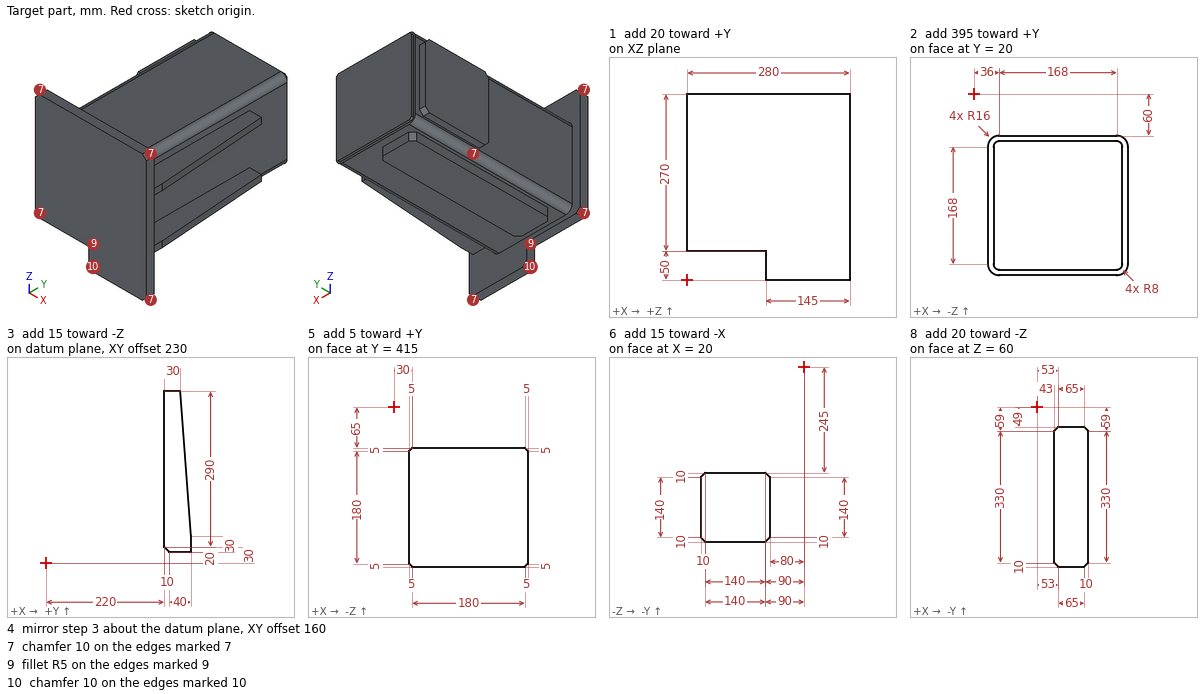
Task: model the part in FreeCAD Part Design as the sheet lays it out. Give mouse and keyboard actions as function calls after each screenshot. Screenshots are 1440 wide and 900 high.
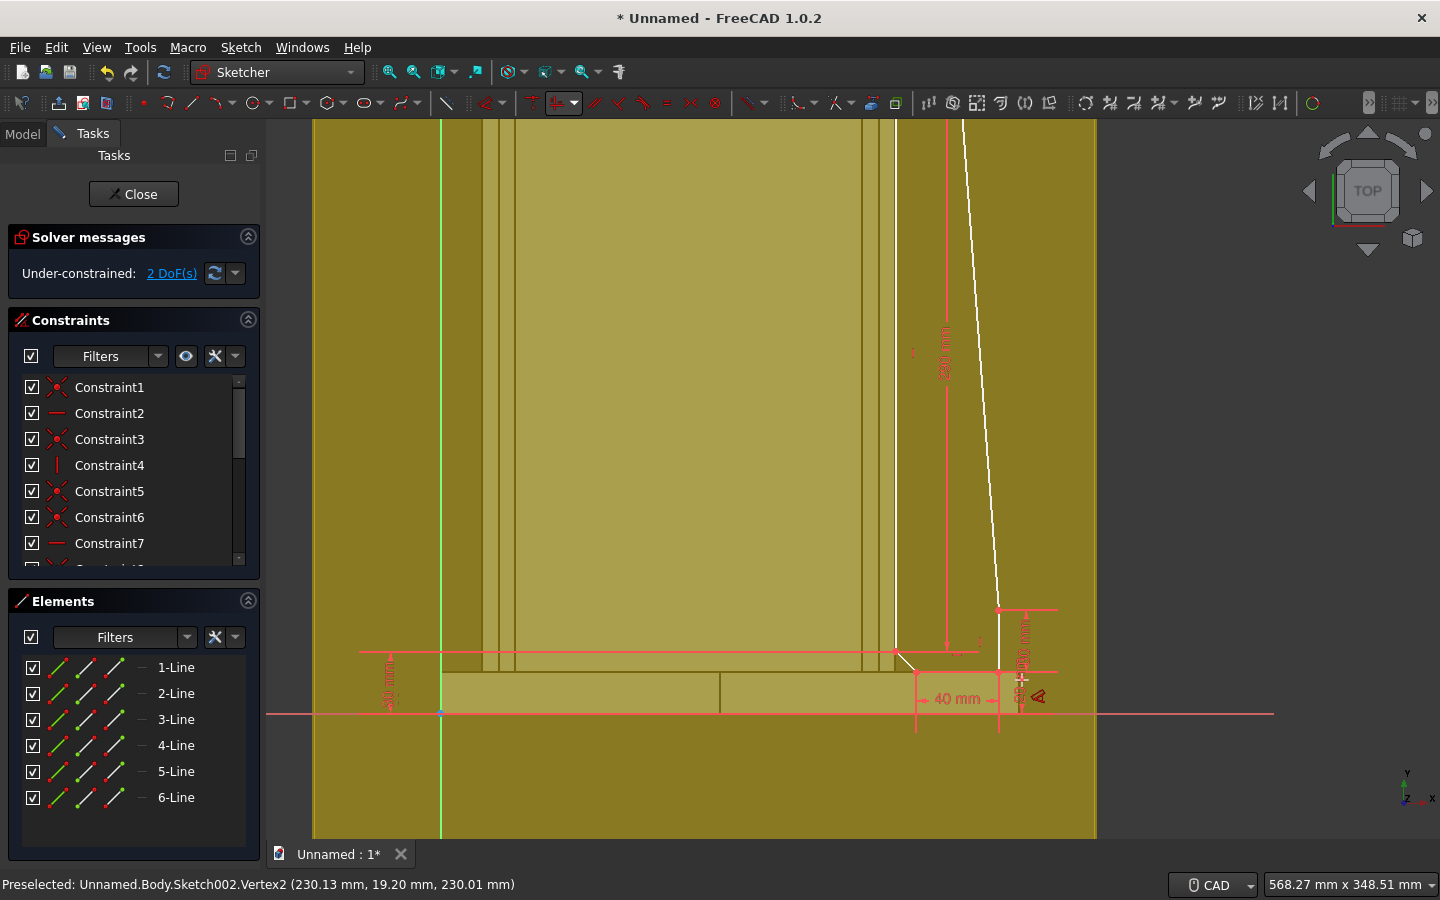
scroll(904, 660, up, 4)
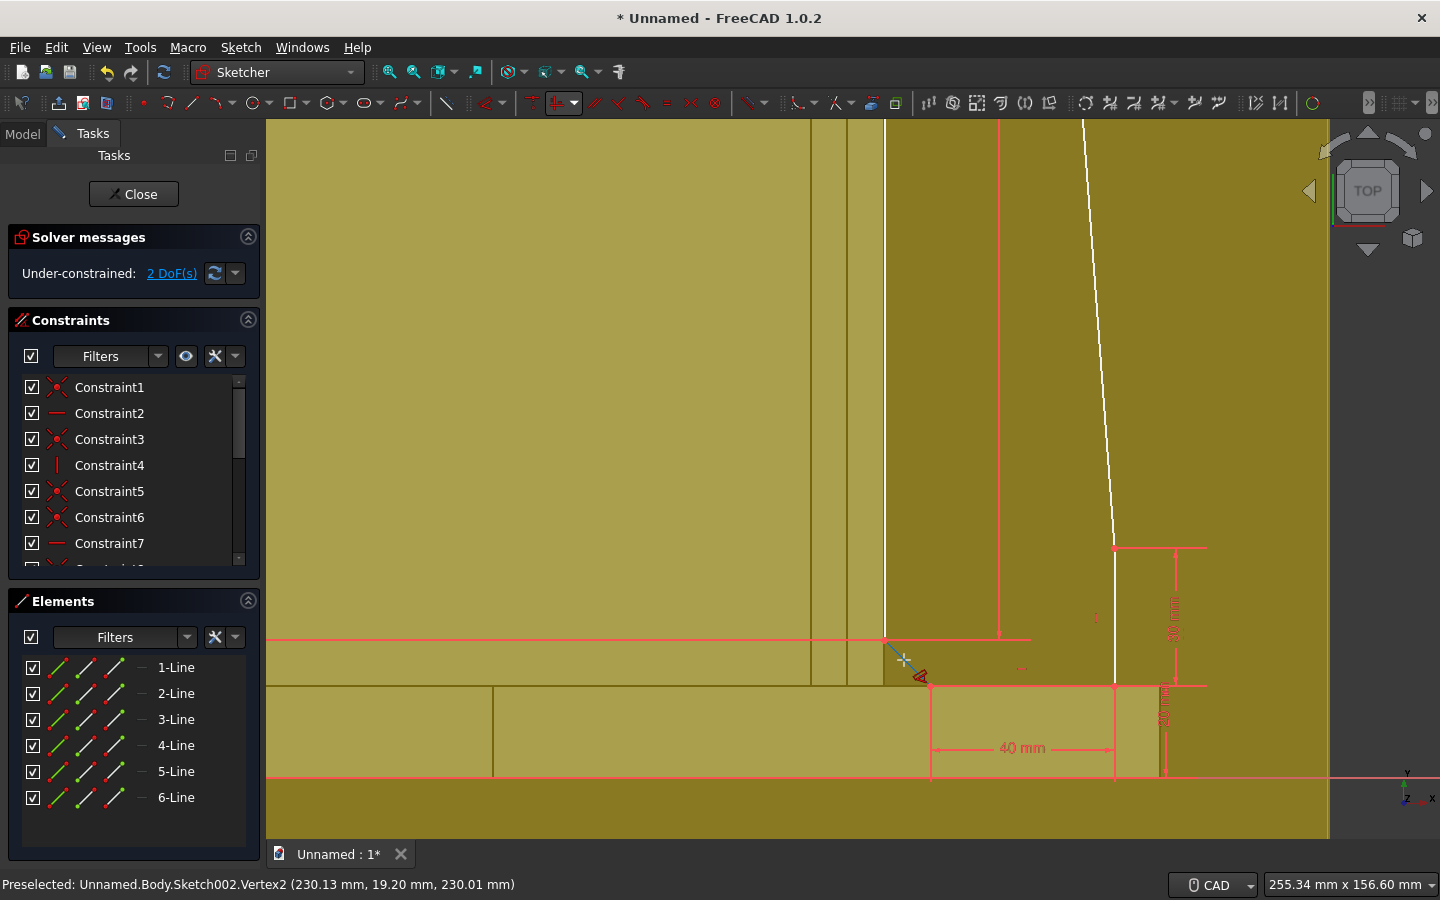
click(903, 659)
click(908, 720)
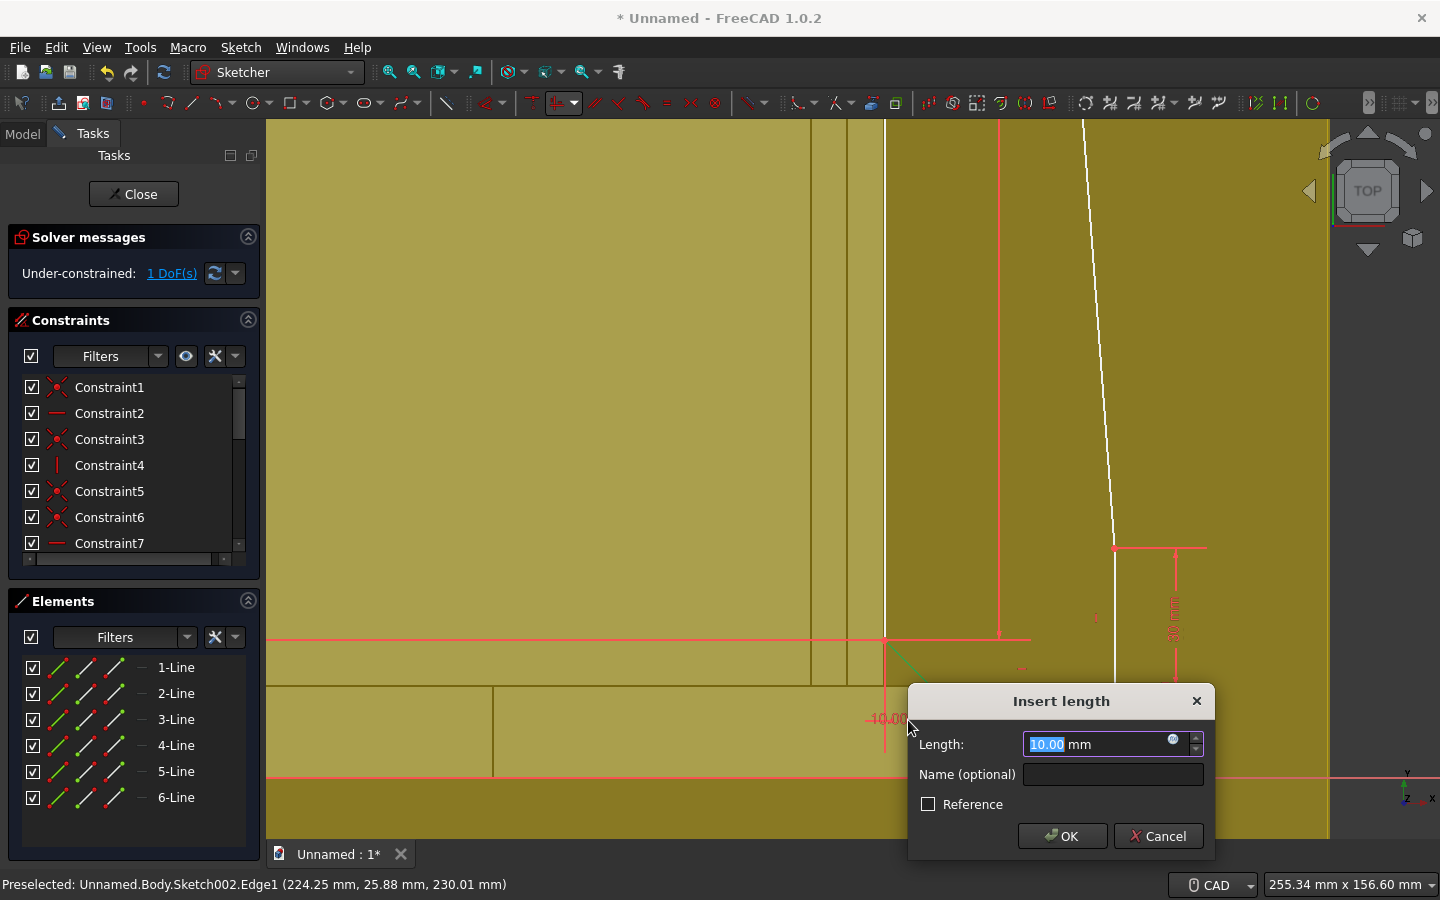
text(10)
key(Return)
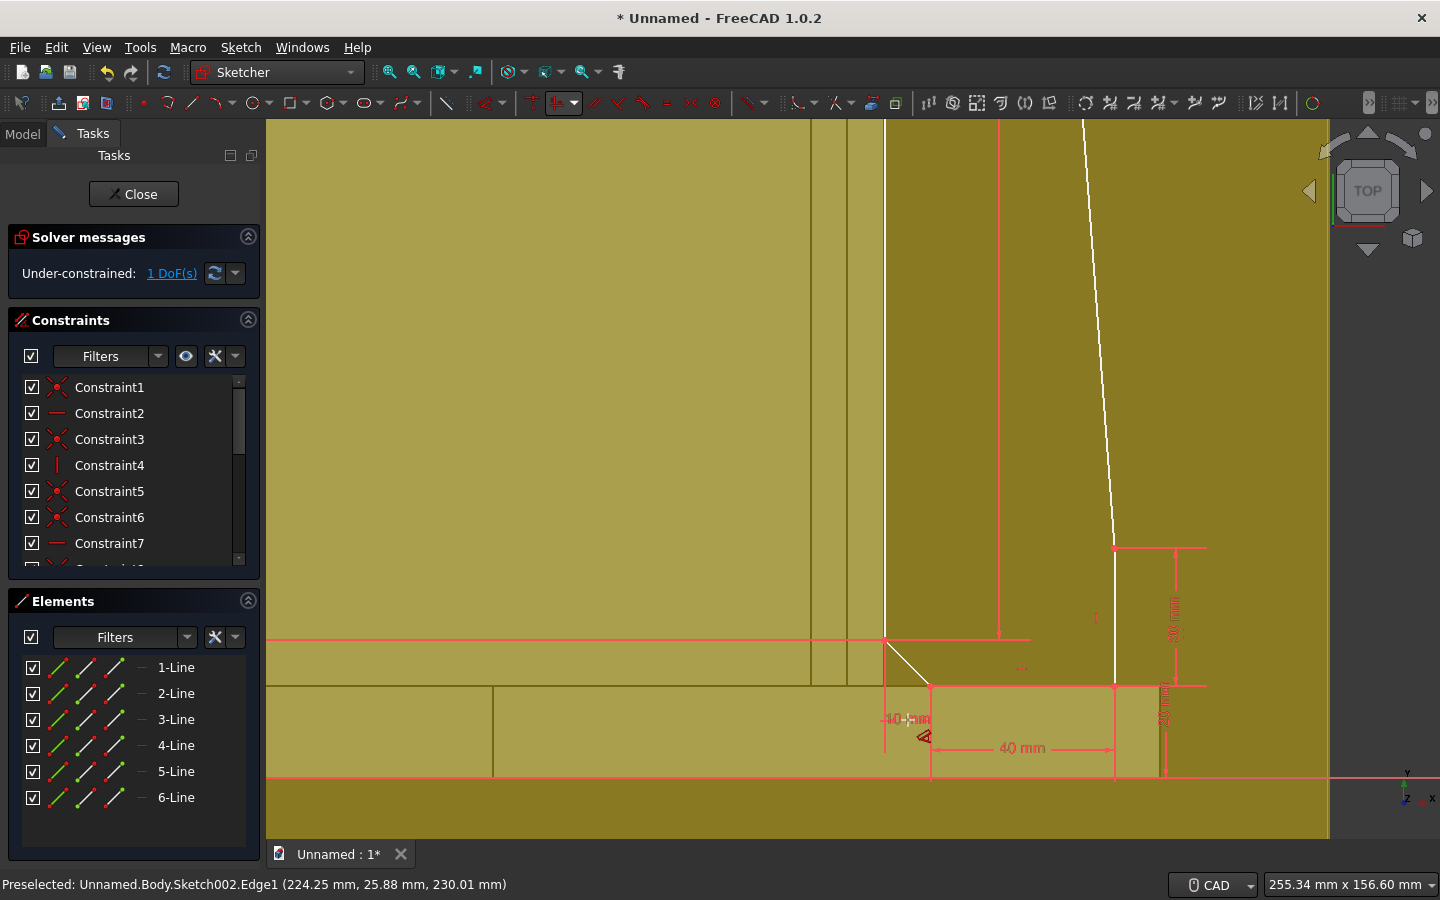
scroll(910, 667, down, 6)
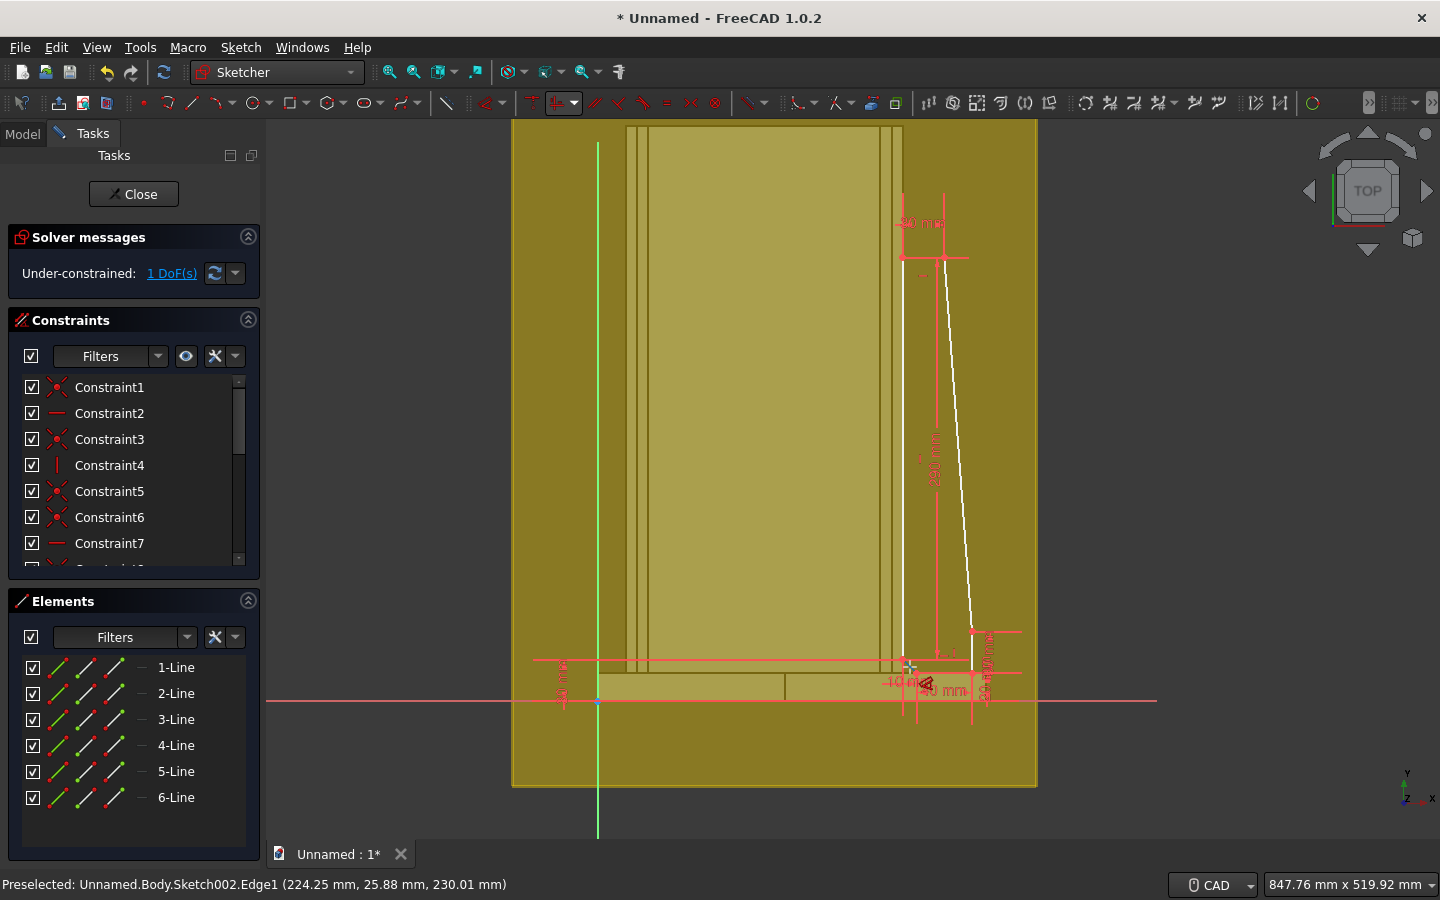
click(903, 660)
click(750, 735)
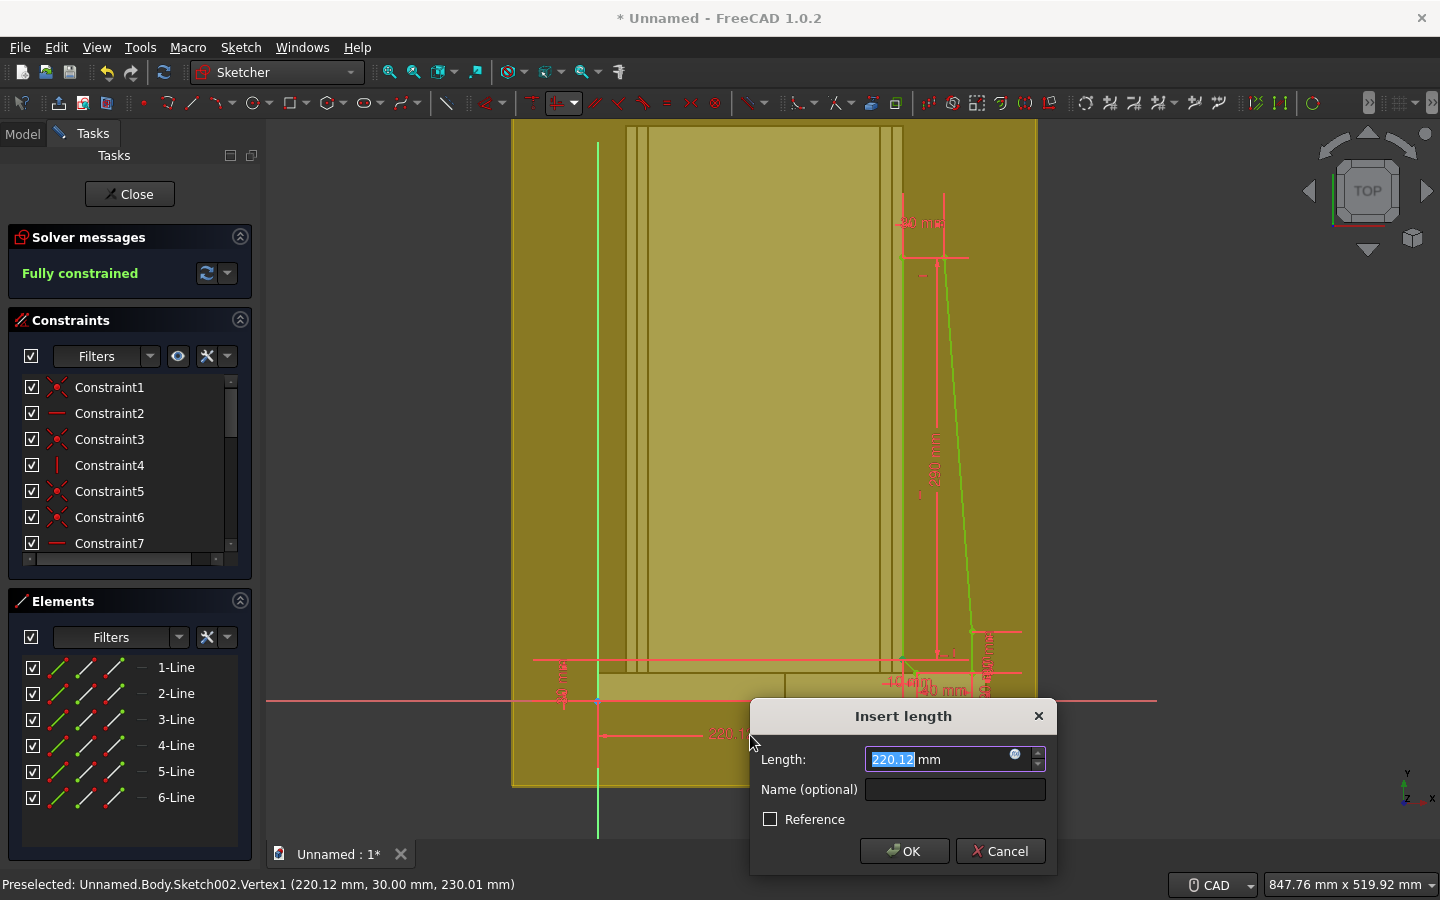
text(220)
key(Return)
key(Escape)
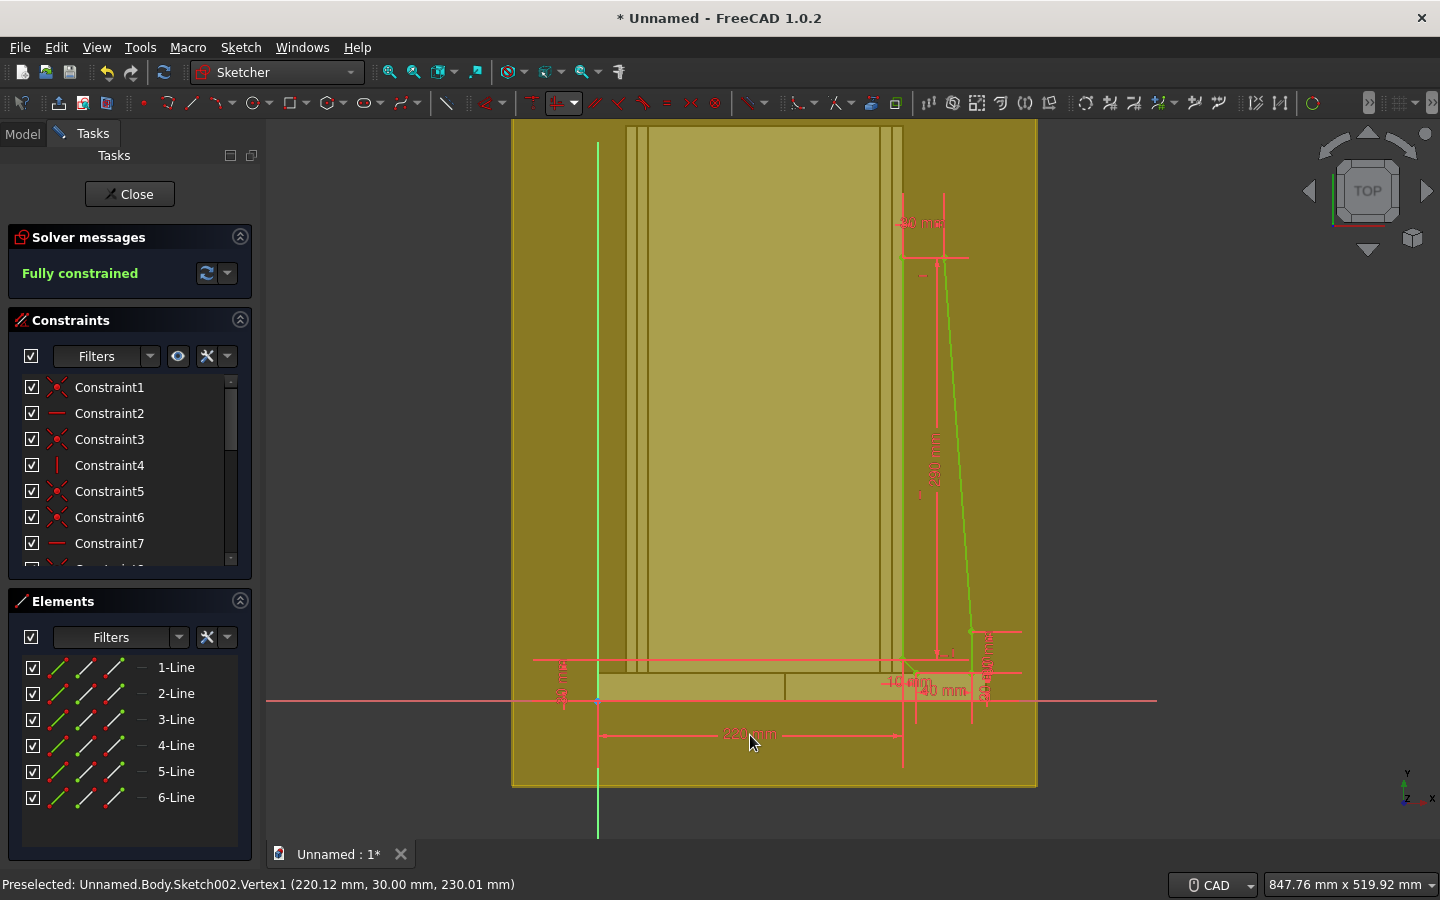
click(130, 194)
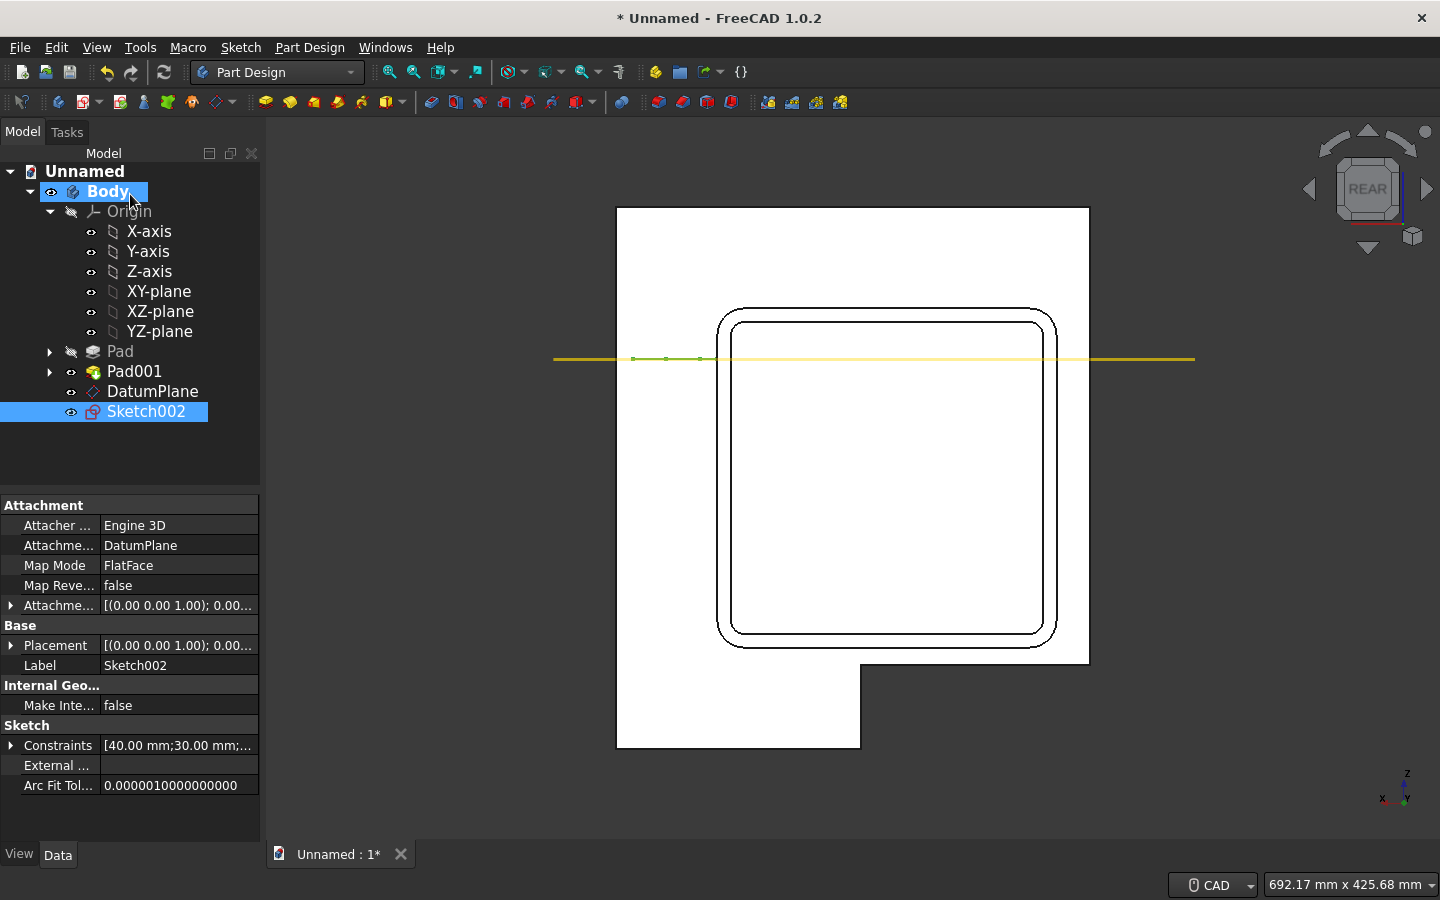
click(266, 102)